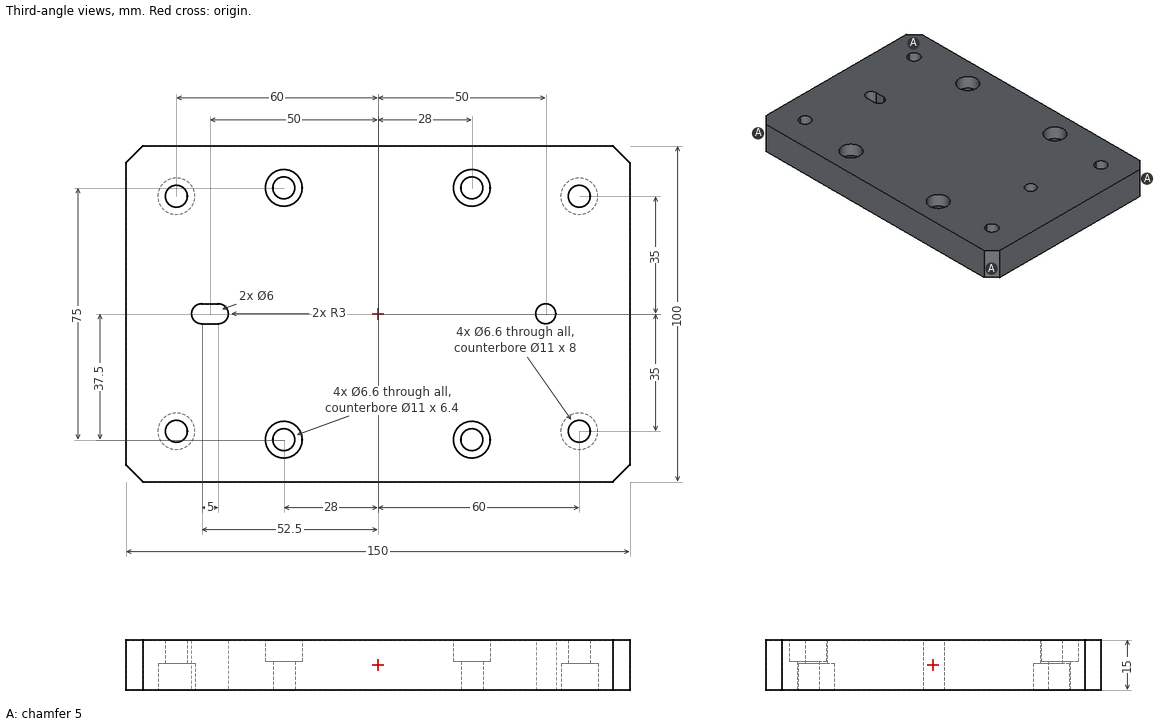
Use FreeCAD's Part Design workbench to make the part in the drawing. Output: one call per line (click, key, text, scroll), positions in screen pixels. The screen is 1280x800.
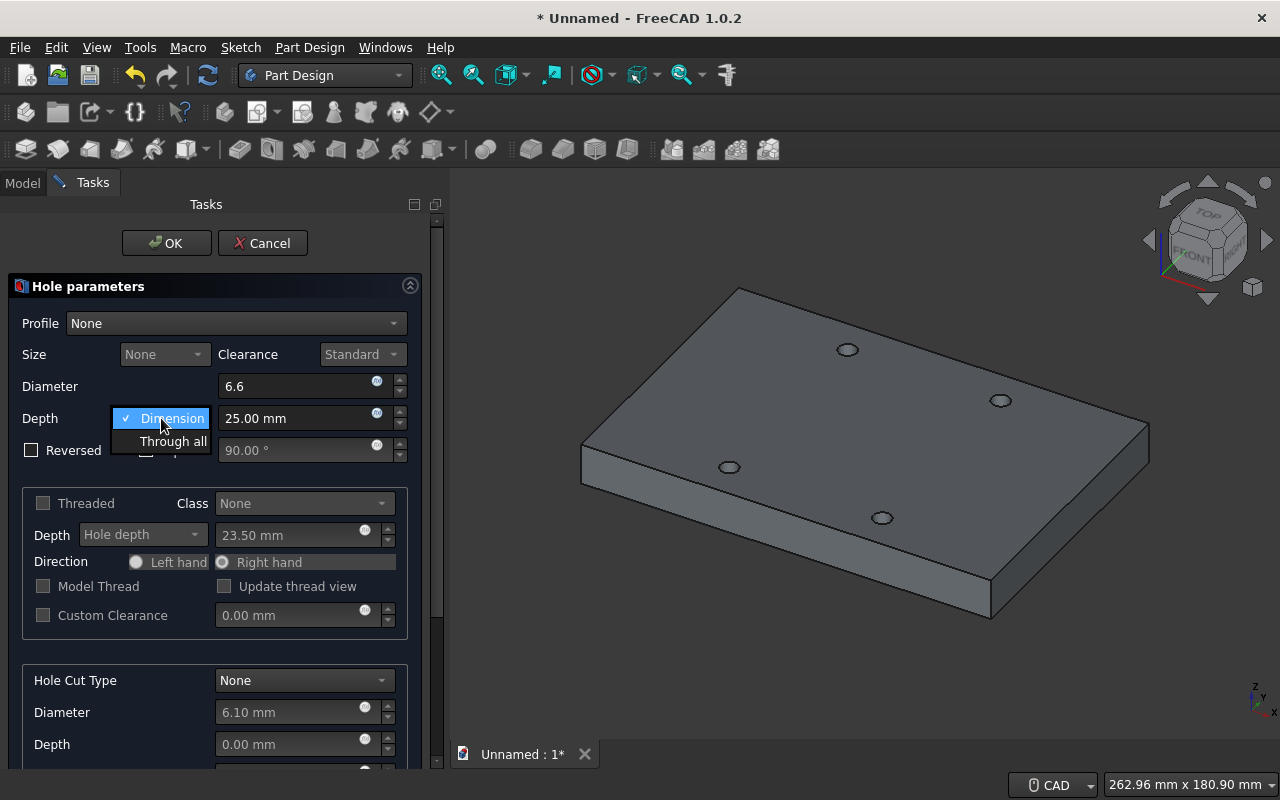
click(160, 442)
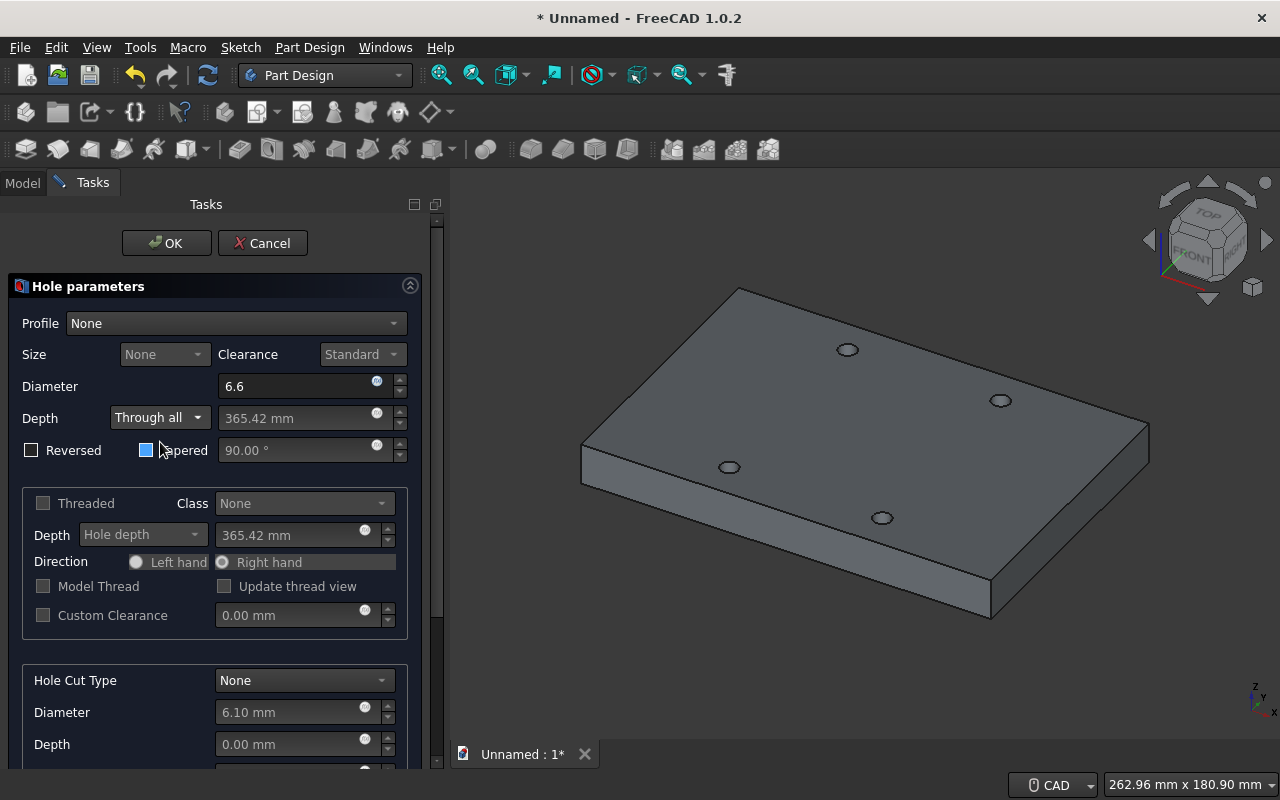
click(306, 680)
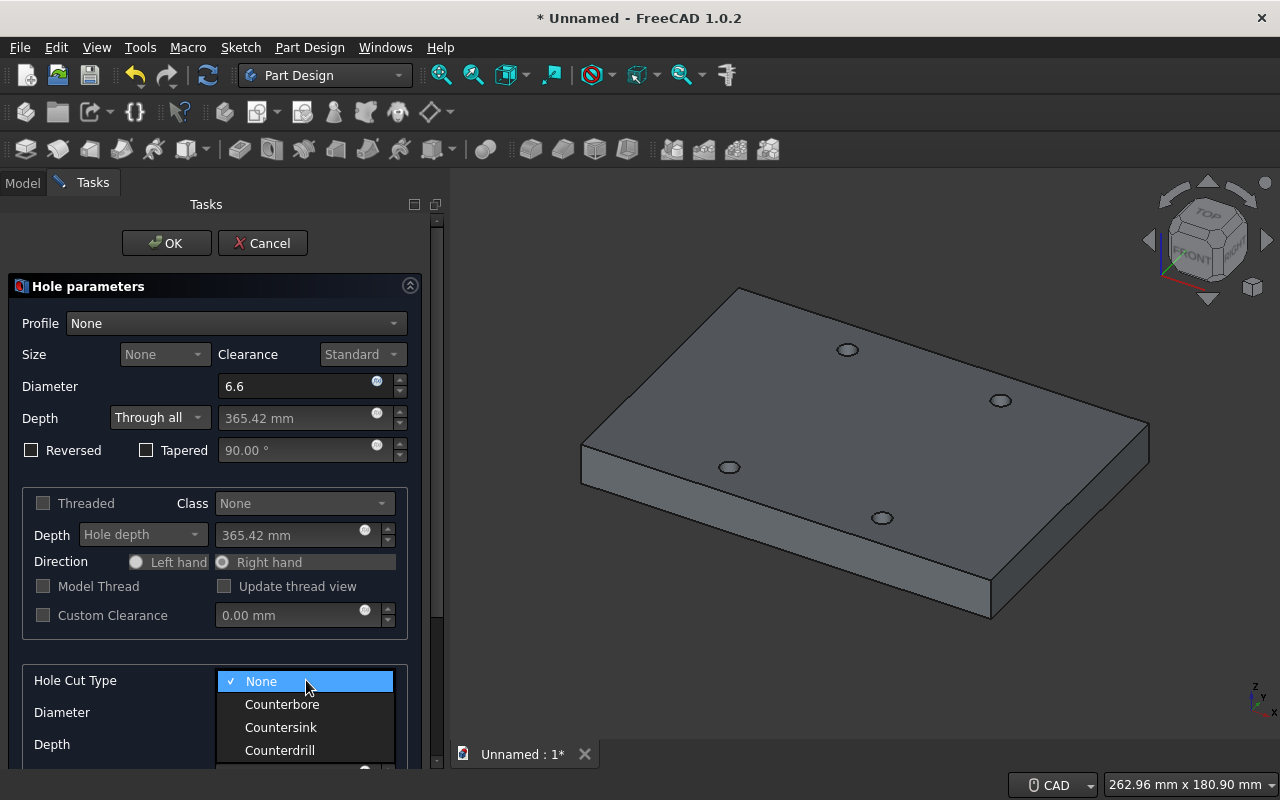
click(304, 704)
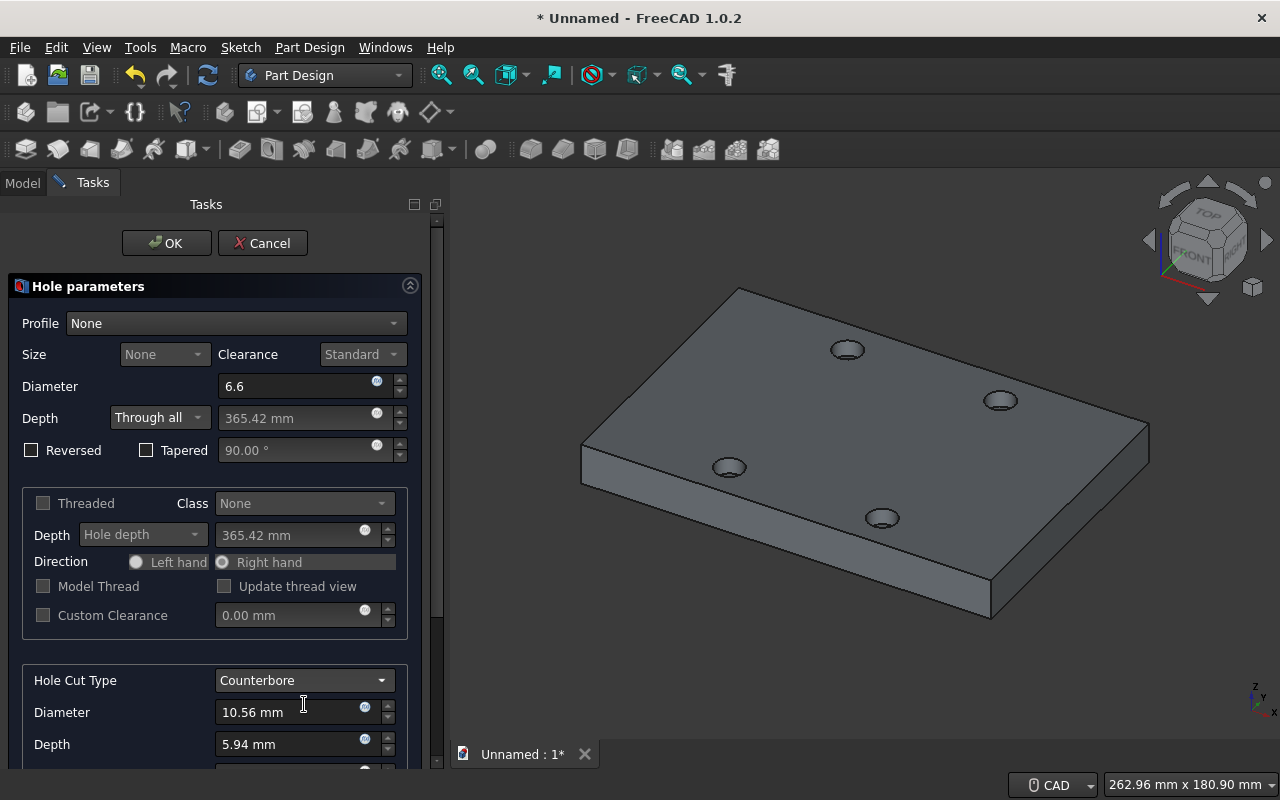
triple_click(298, 712)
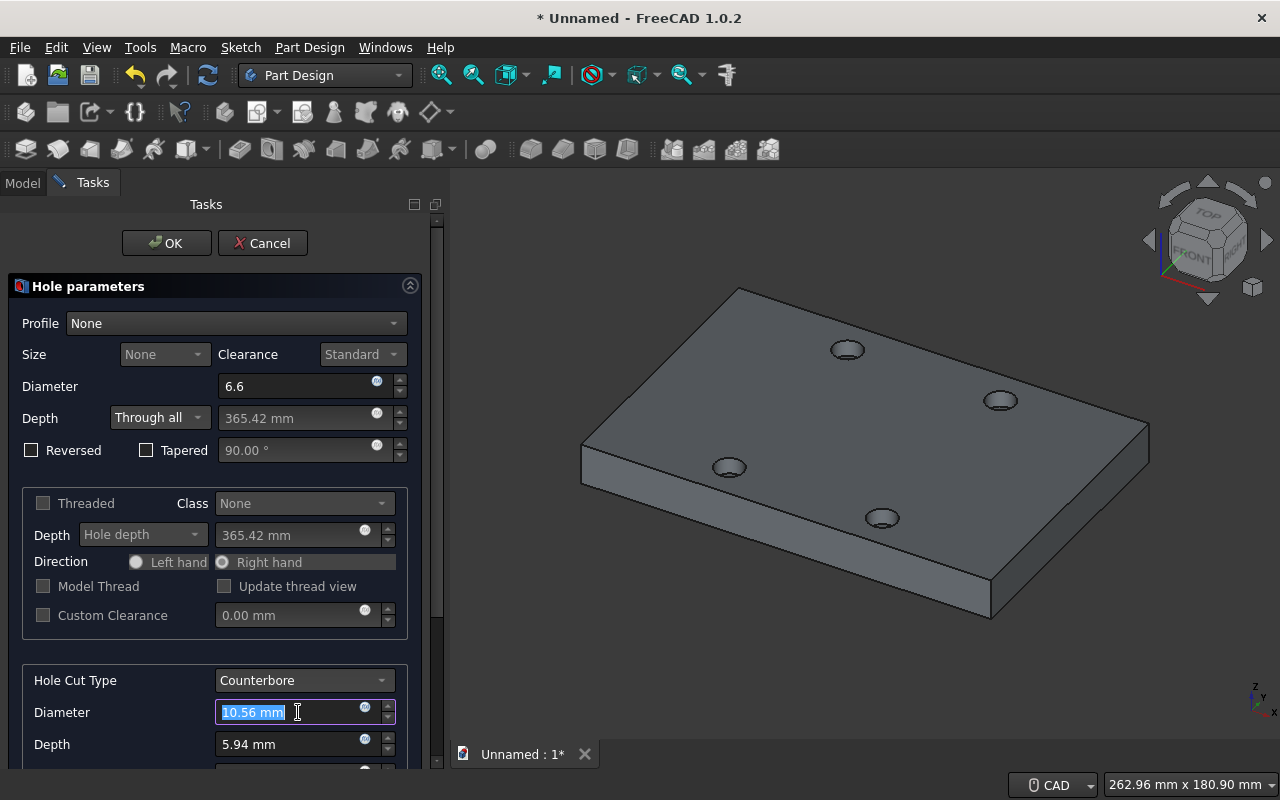
text(11)
key(Tab)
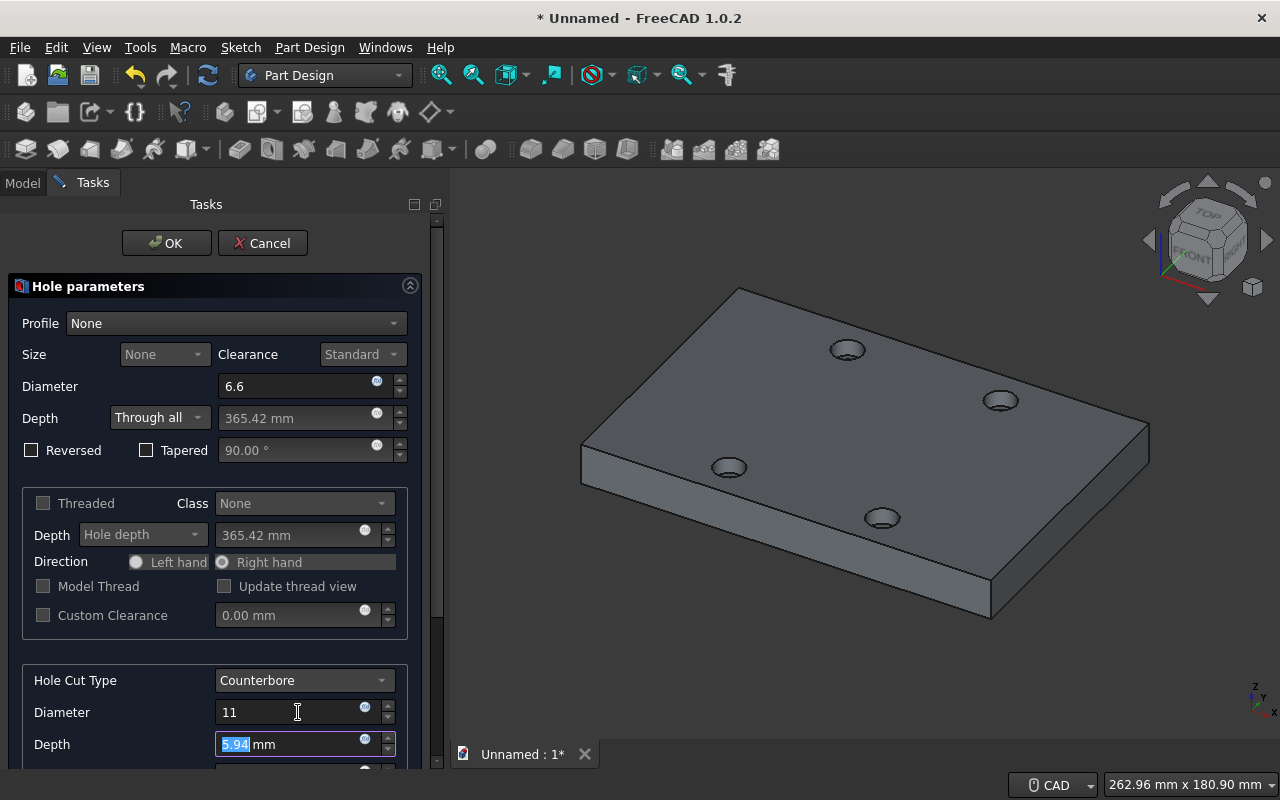
text(6.4)
key(Tab)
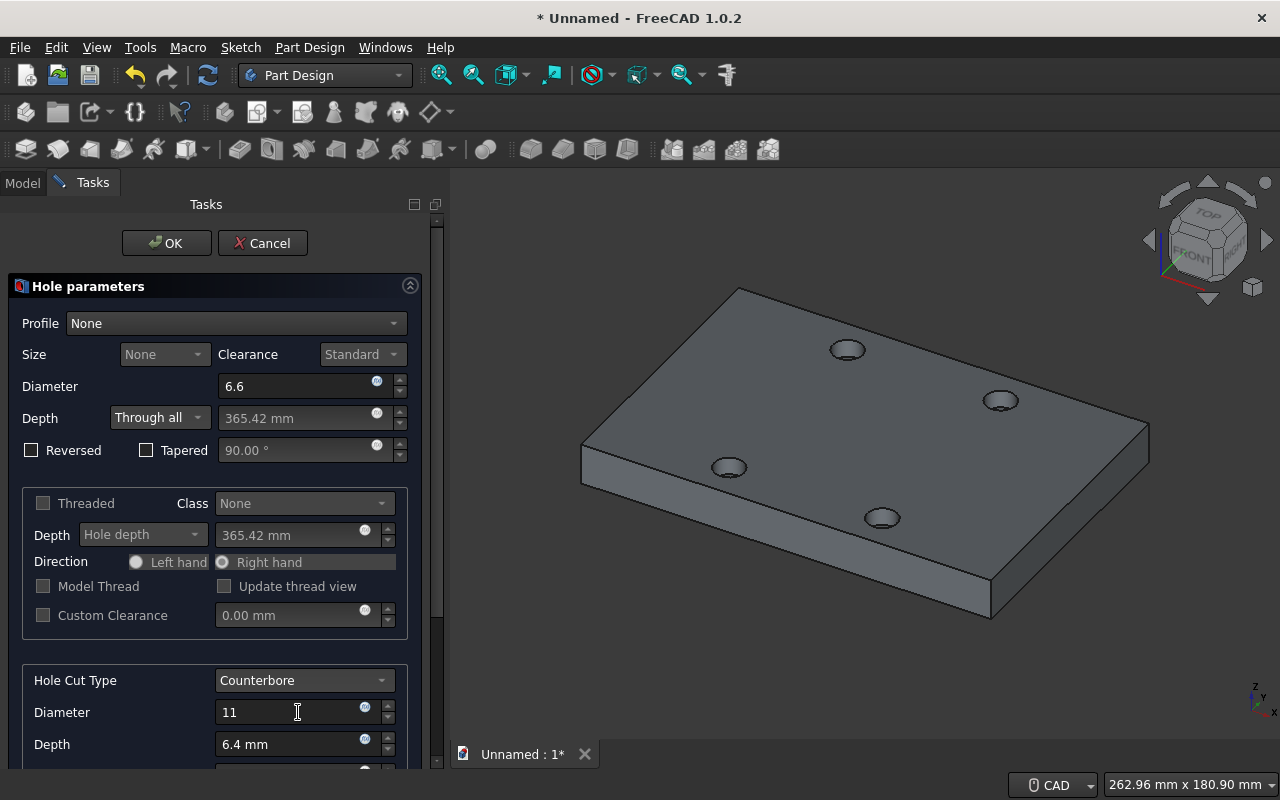
click(167, 243)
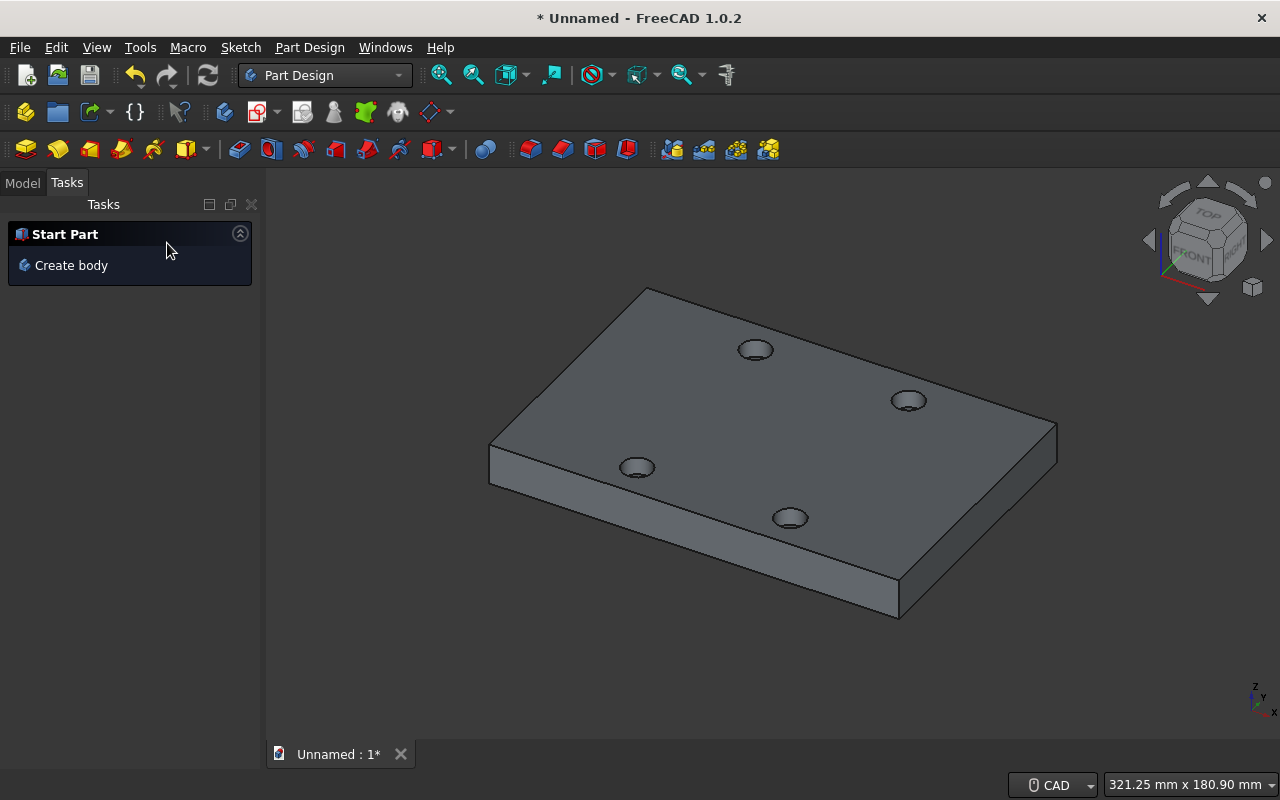
click(899, 599)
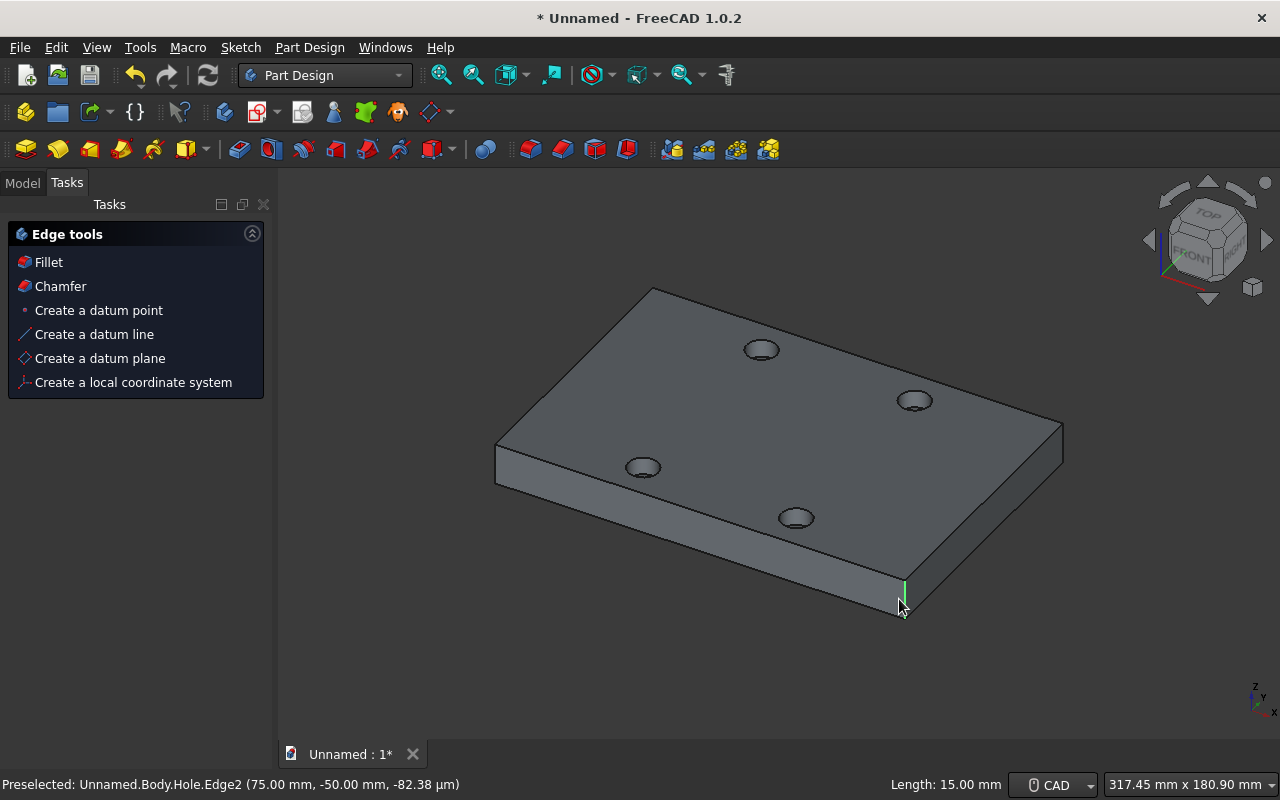
key(0)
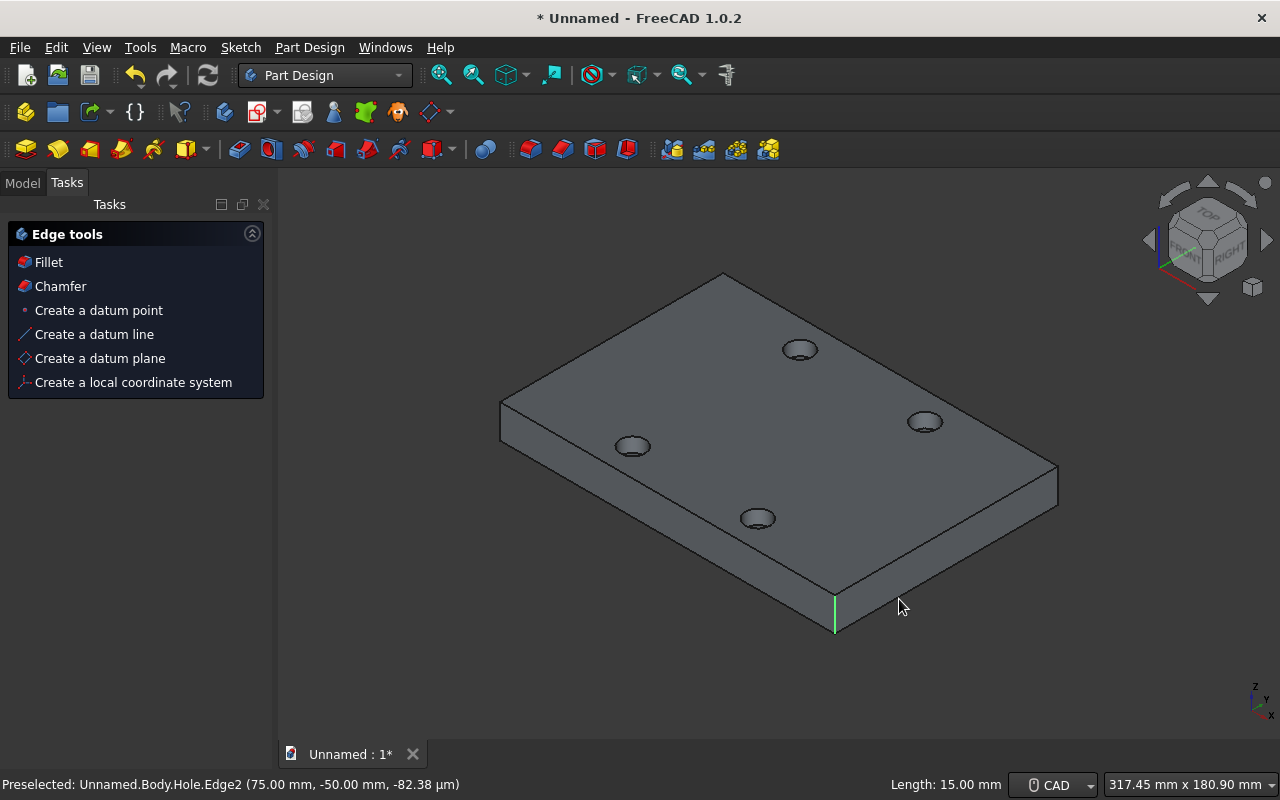
key(2)